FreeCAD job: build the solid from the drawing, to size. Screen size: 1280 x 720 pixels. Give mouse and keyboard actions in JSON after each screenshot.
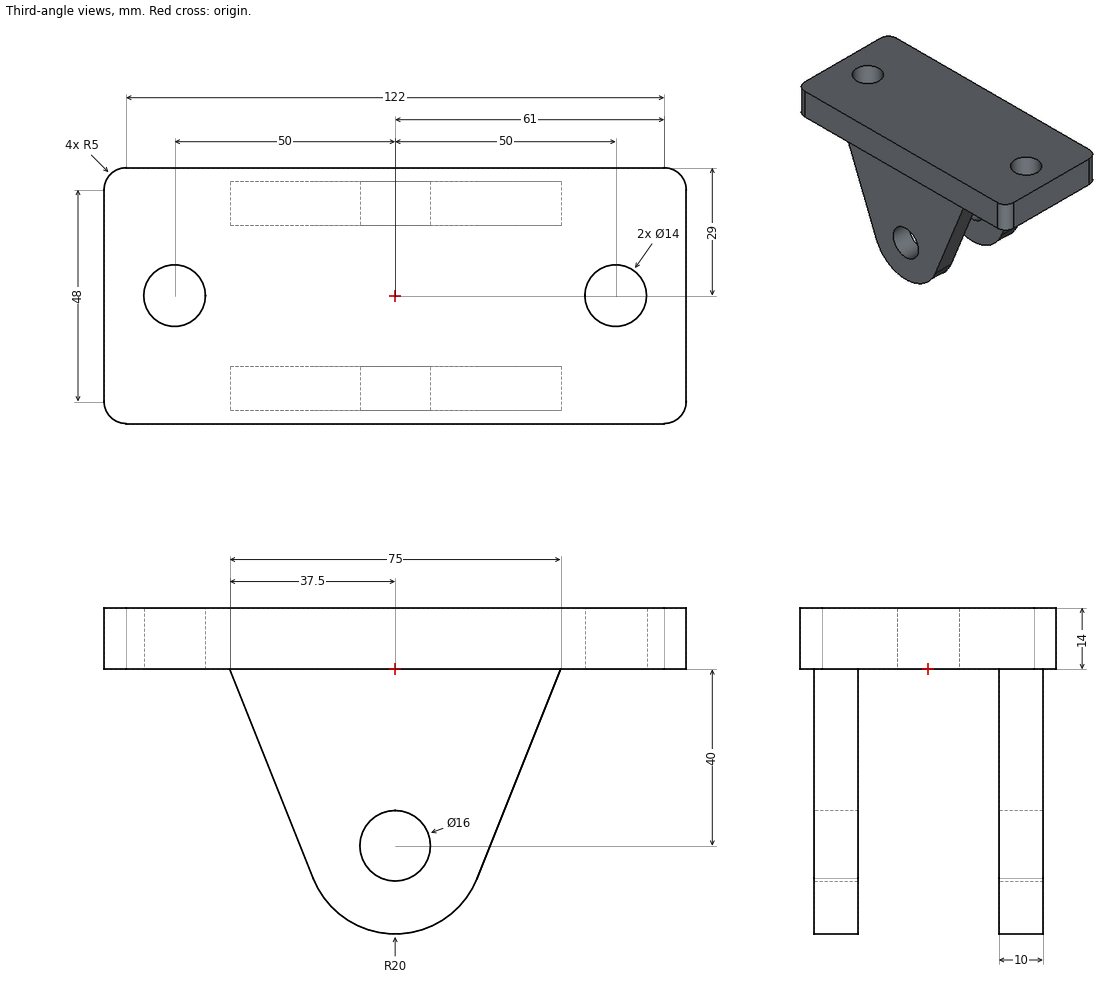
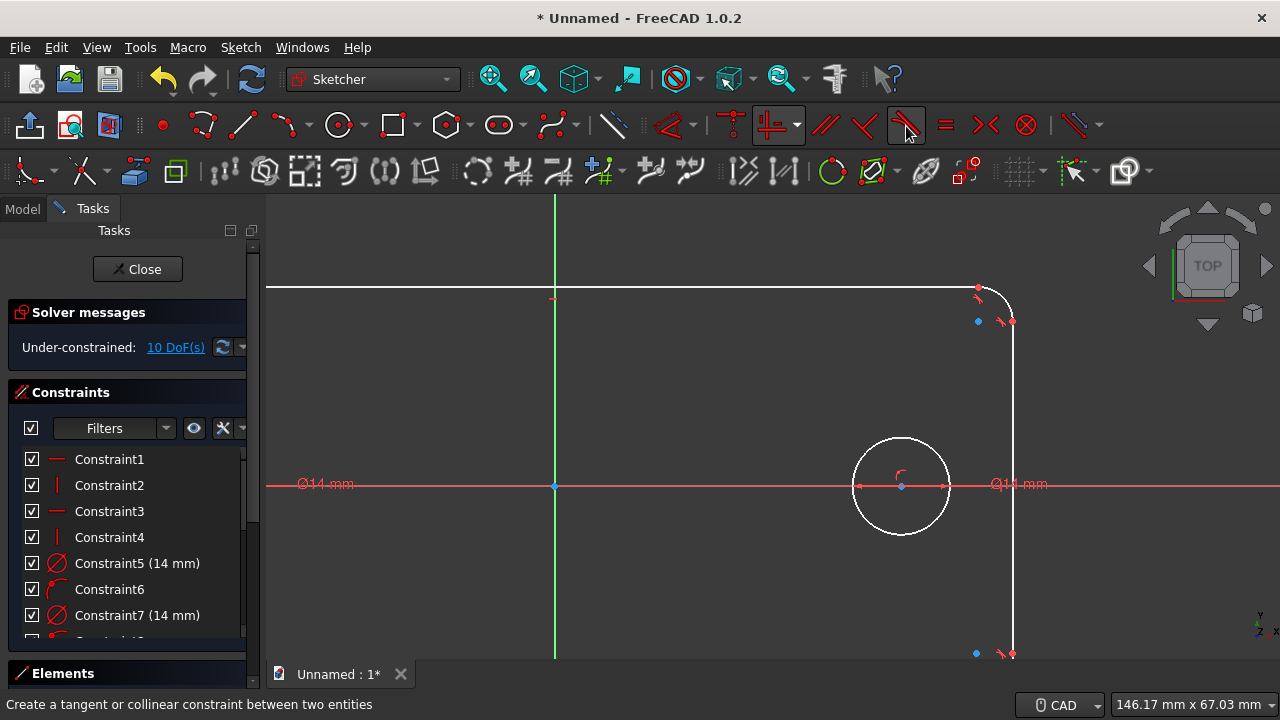
{"action": "scroll", "coordinate": [1009, 305], "scroll_direction": "down", "scroll_amount": 2}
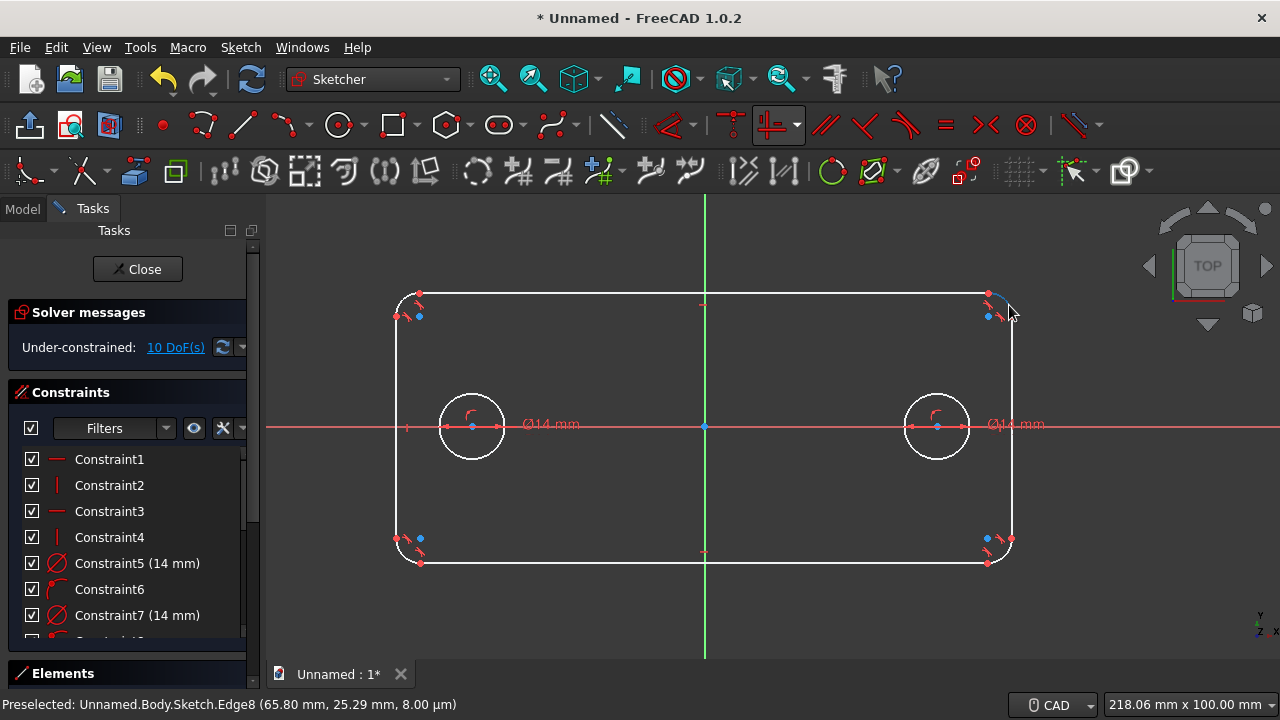
{"action": "scroll", "coordinate": [409, 296], "scroll_direction": "up", "scroll_amount": 2}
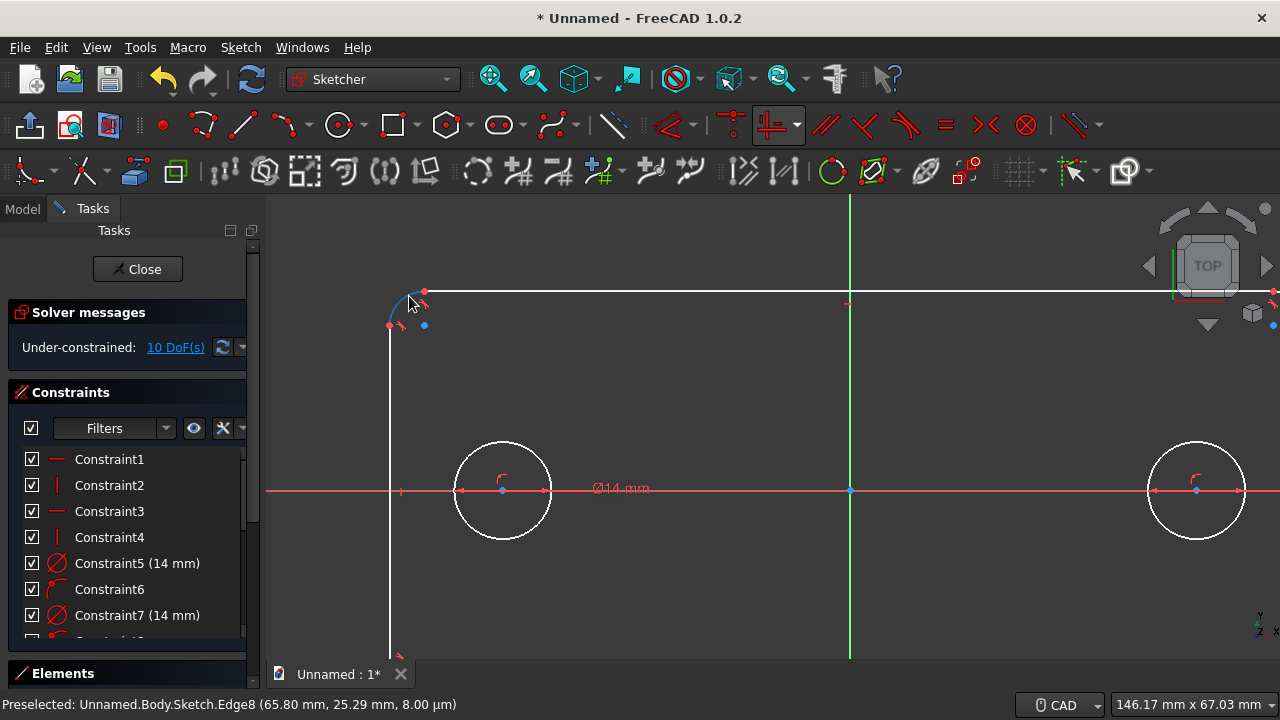
{"action": "left_click", "coordinate": [409, 295]}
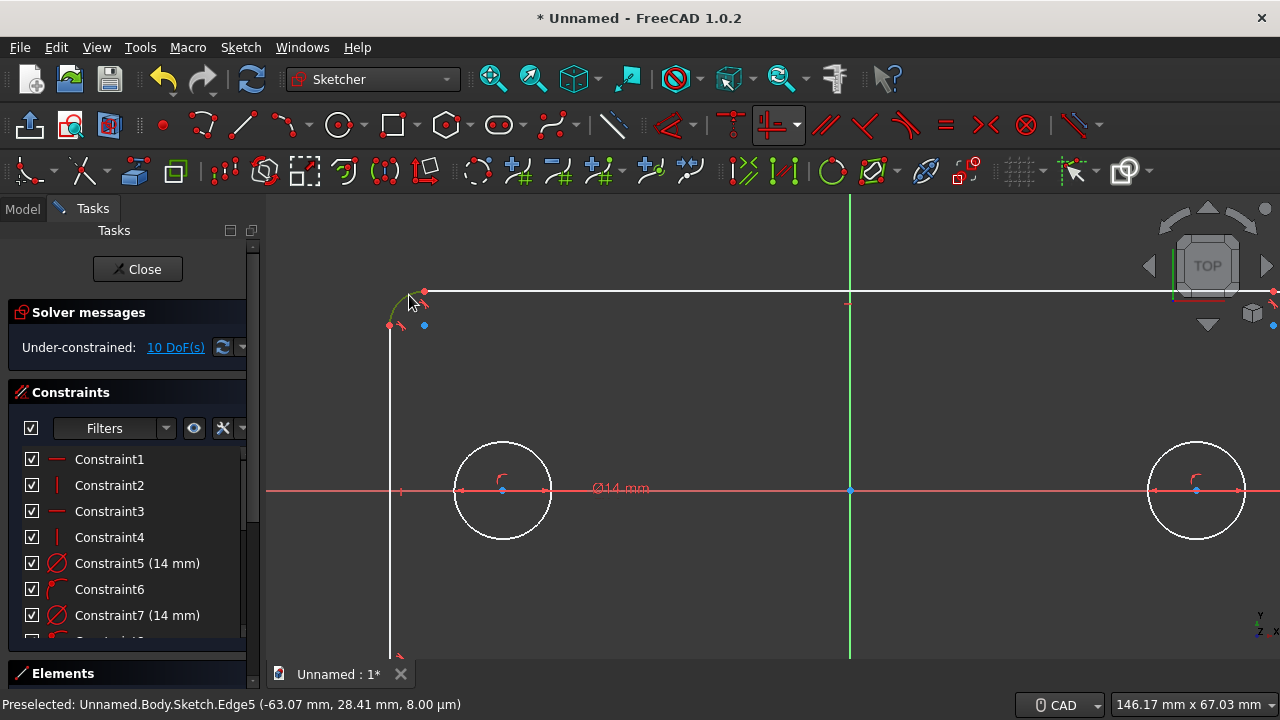
{"action": "scroll", "coordinate": [409, 296], "scroll_direction": "down", "scroll_amount": 2}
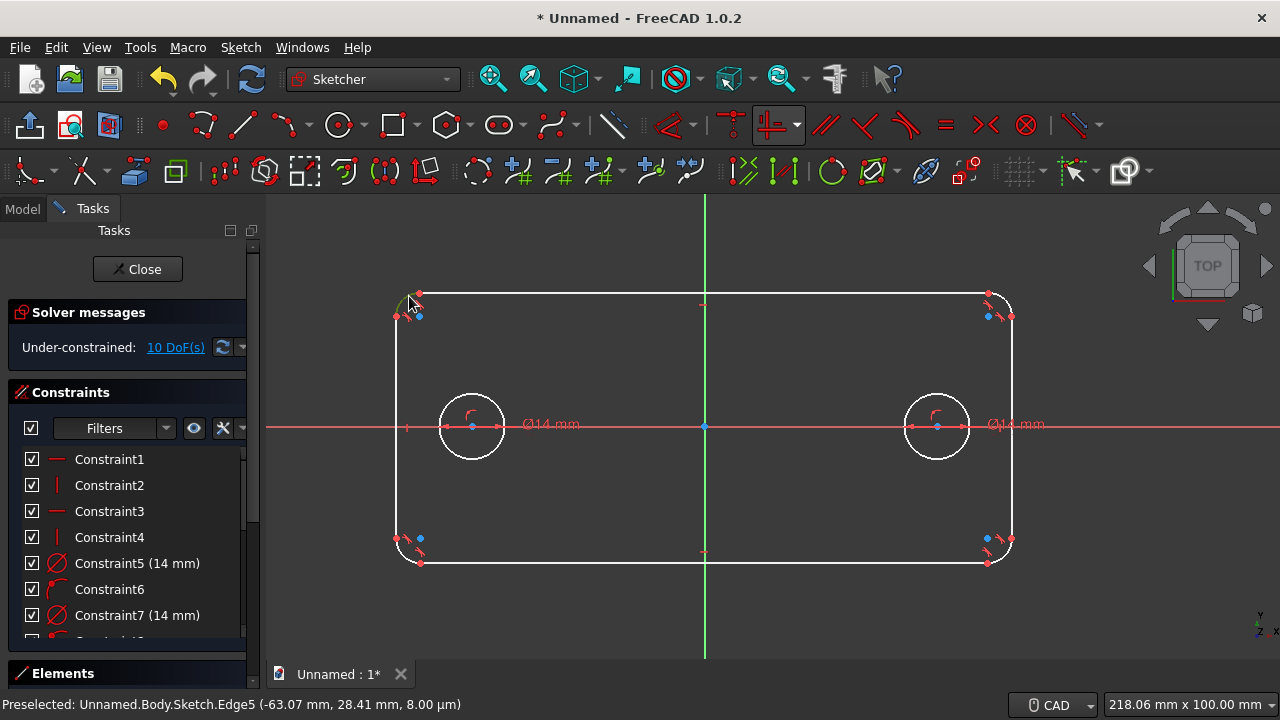
{"action": "left_click", "coordinate": [399, 550]}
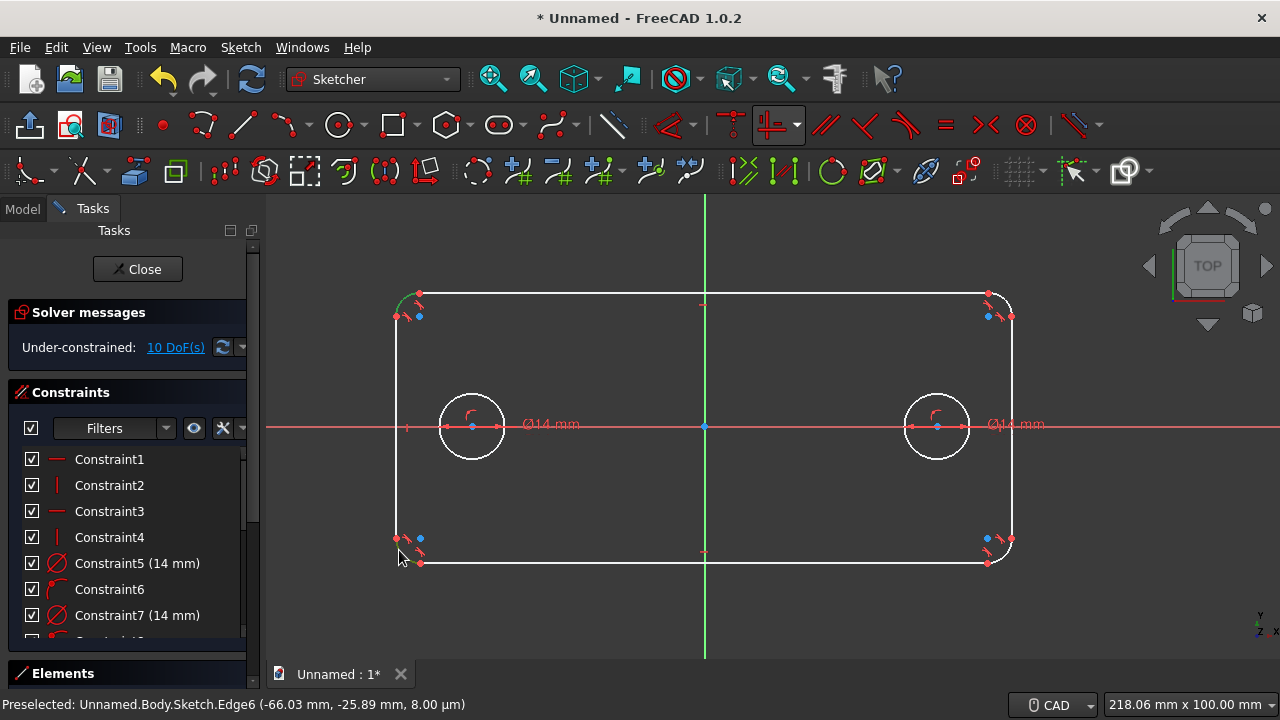
{"action": "left_click", "coordinate": [999, 560]}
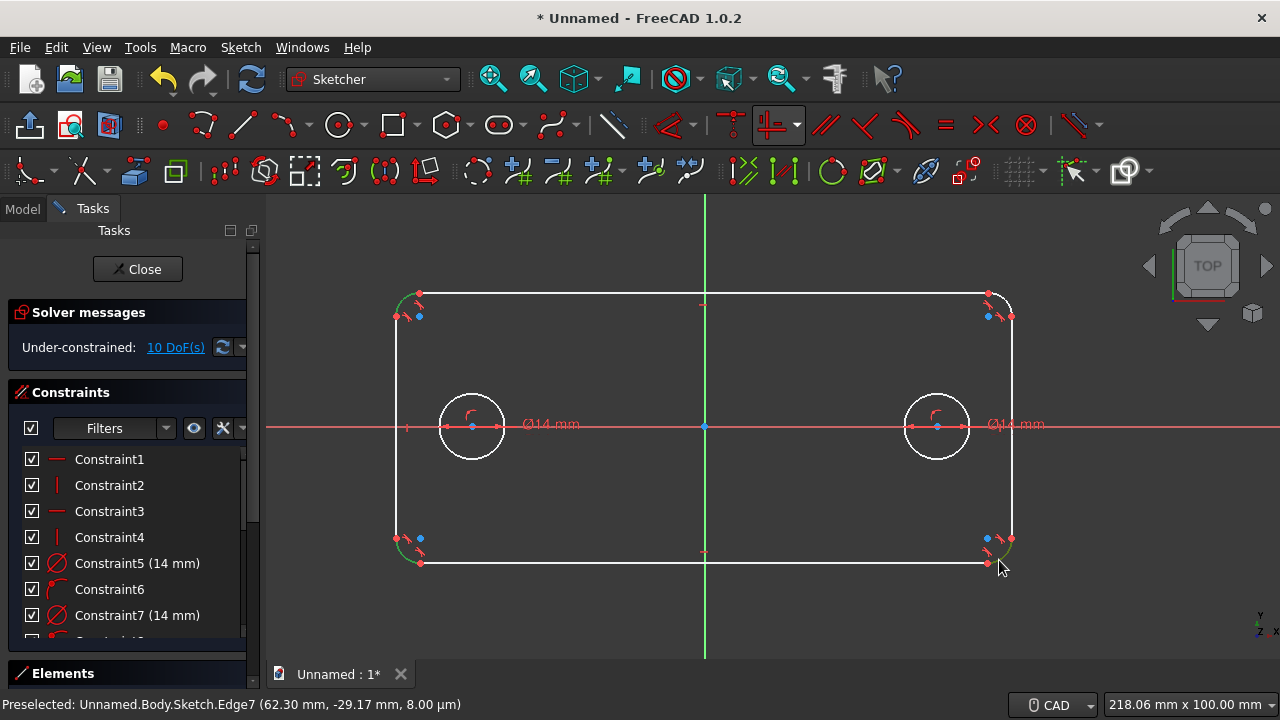
{"action": "scroll", "coordinate": [1009, 306], "scroll_direction": "up", "scroll_amount": 2}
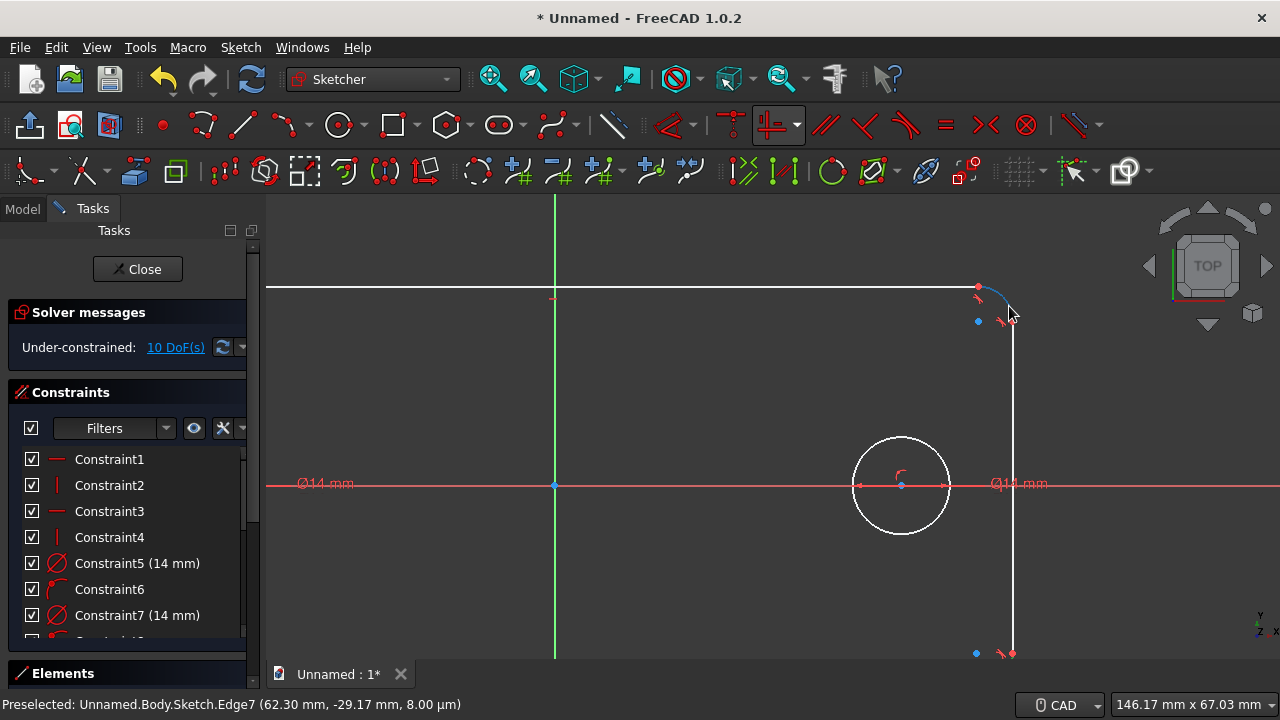
{"action": "left_click", "coordinate": [1009, 305]}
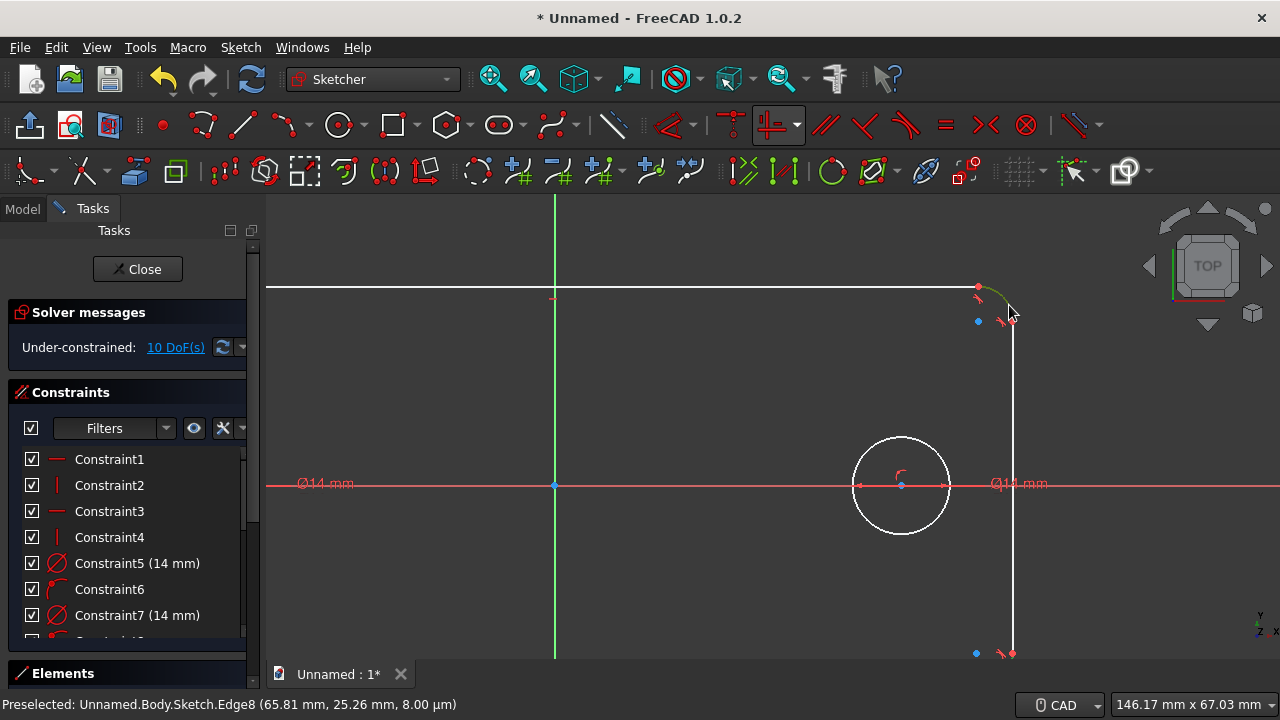
{"action": "left_click", "coordinate": [946, 126]}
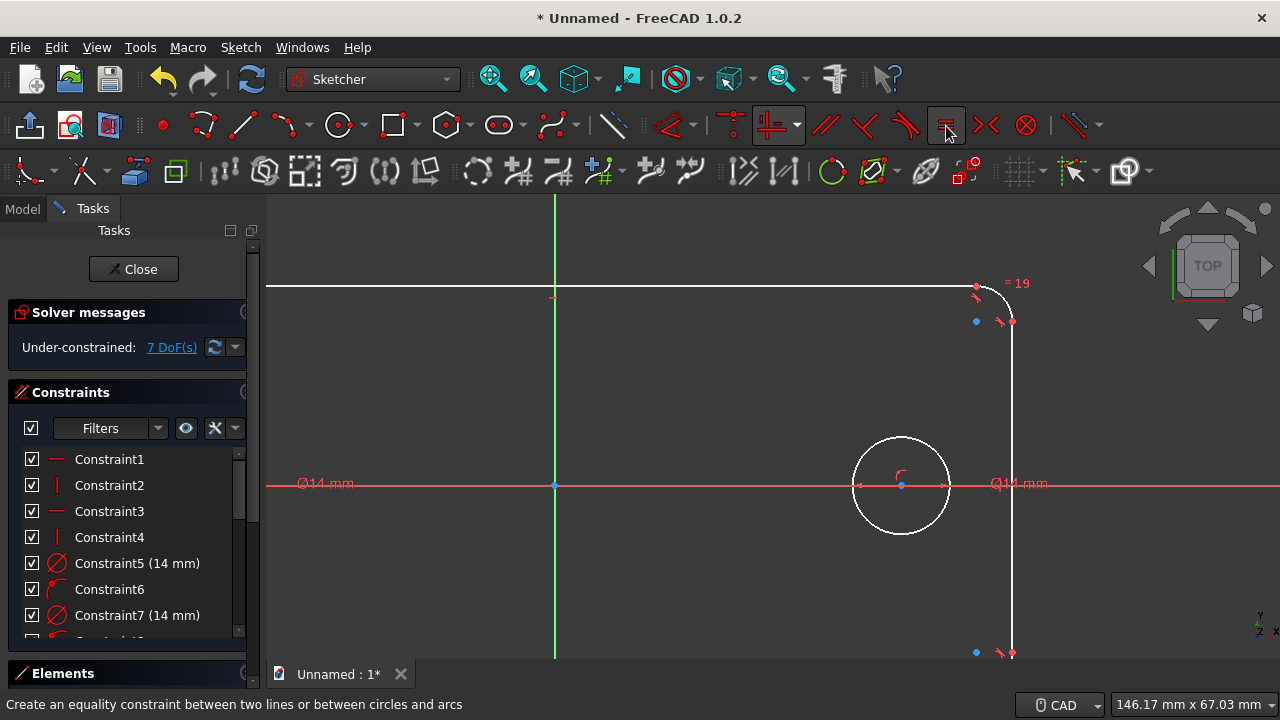
{"action": "left_click", "coordinate": [668, 126]}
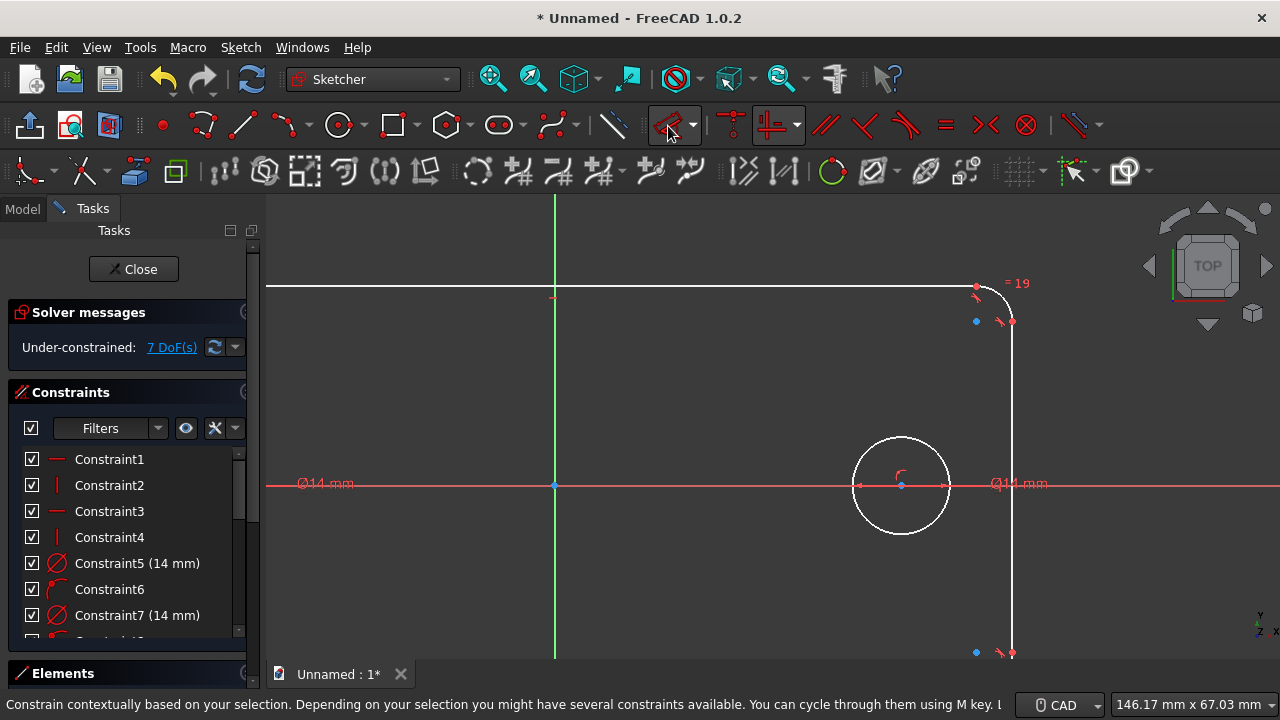
{"action": "scroll", "coordinate": [1009, 306], "scroll_direction": "down", "scroll_amount": 2}